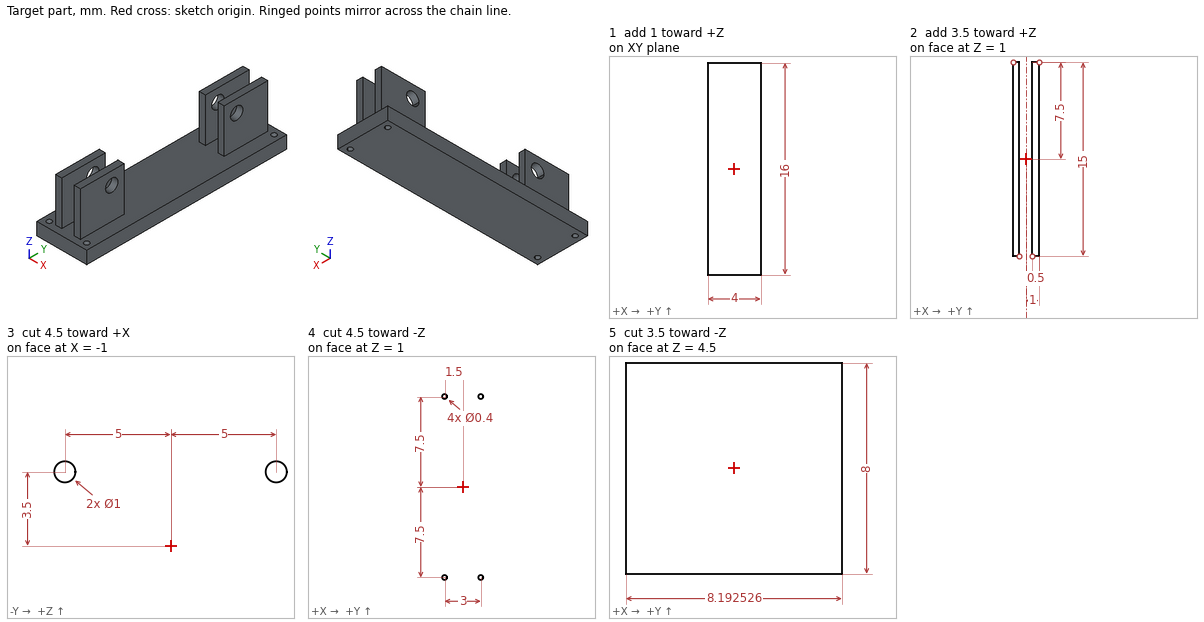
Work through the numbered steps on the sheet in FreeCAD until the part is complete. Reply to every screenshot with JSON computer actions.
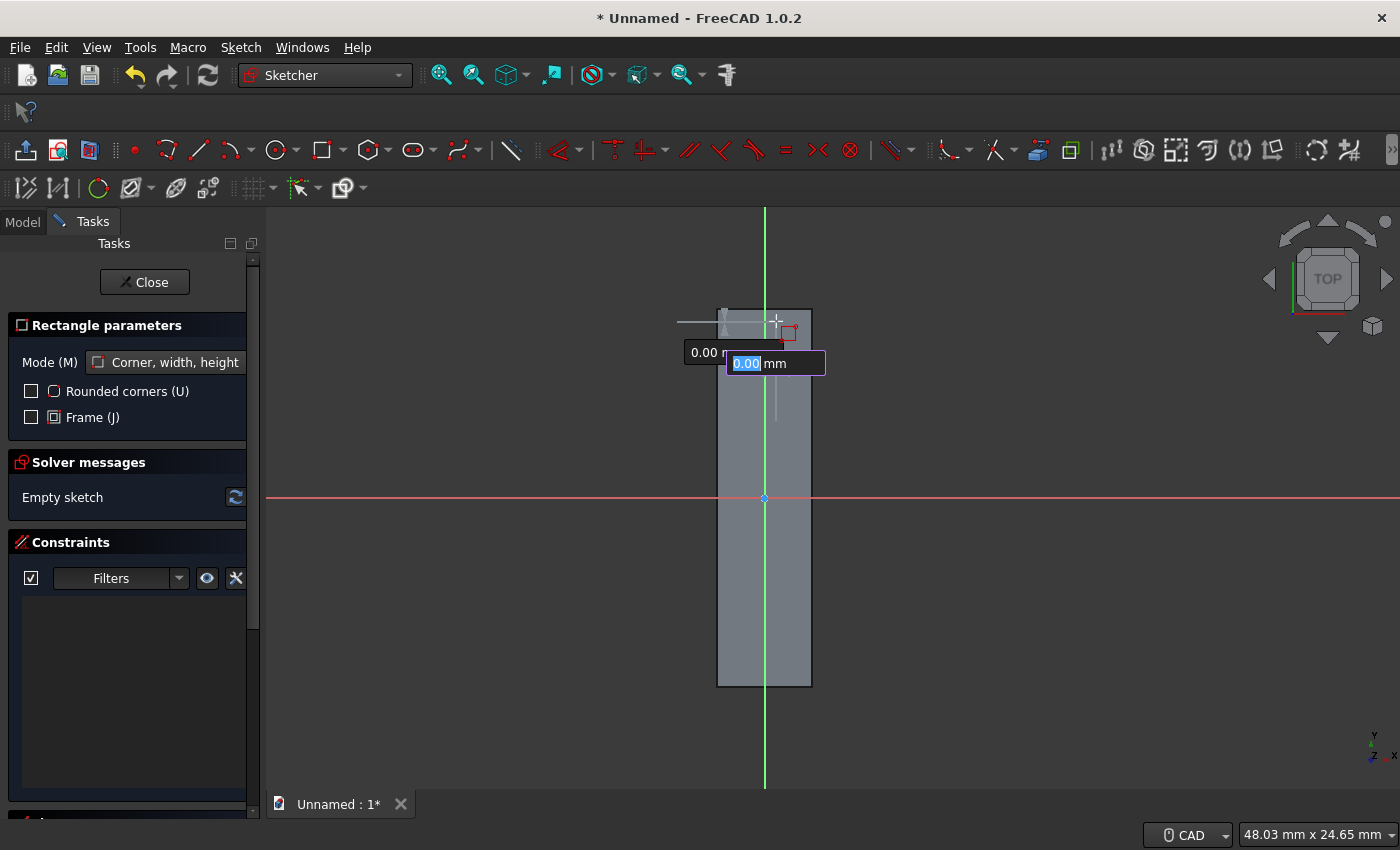
{"action": "left_click", "coordinate": [788, 675]}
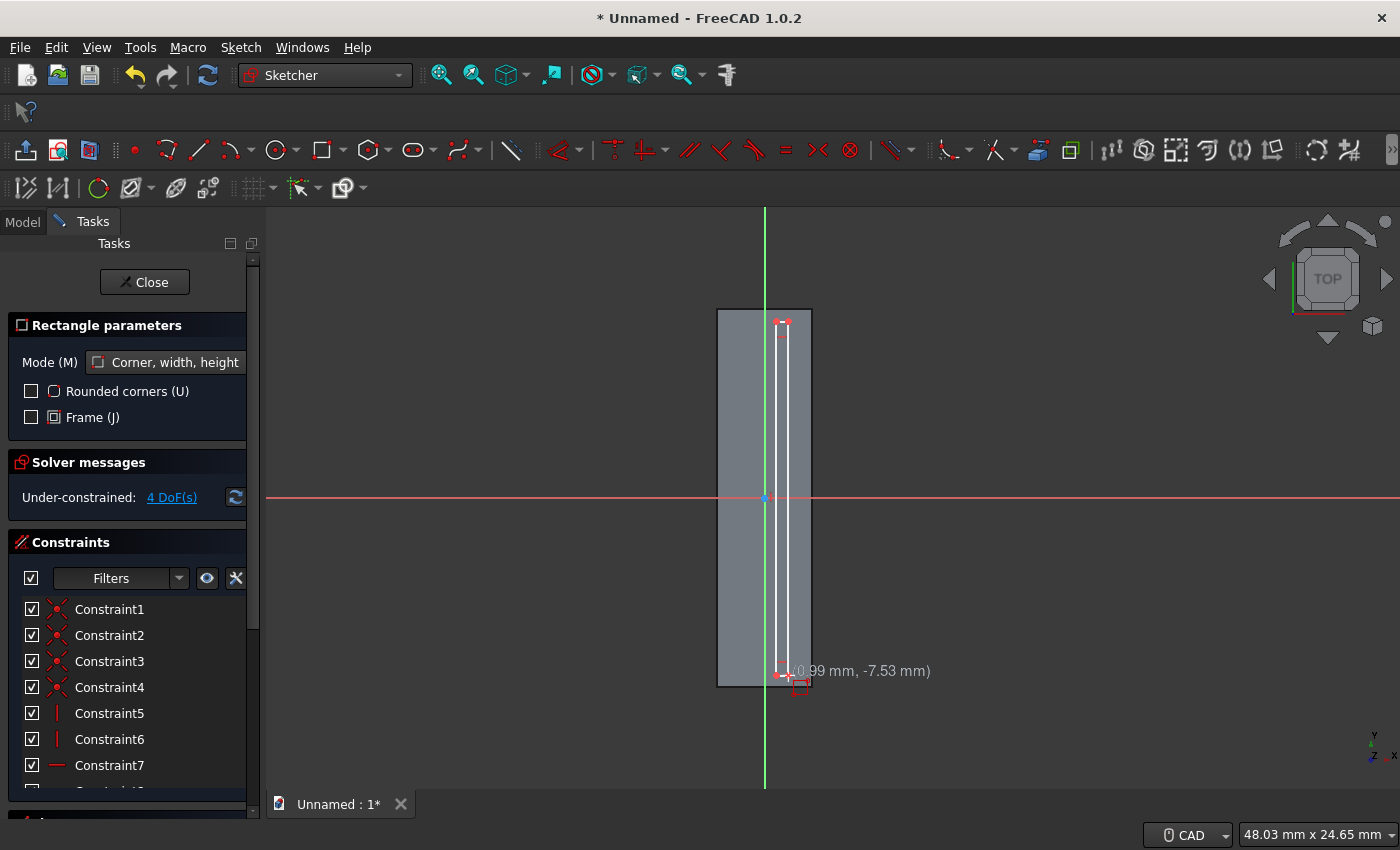
{"action": "scroll", "coordinate": [741, 321], "scroll_direction": "up", "scroll_amount": 2}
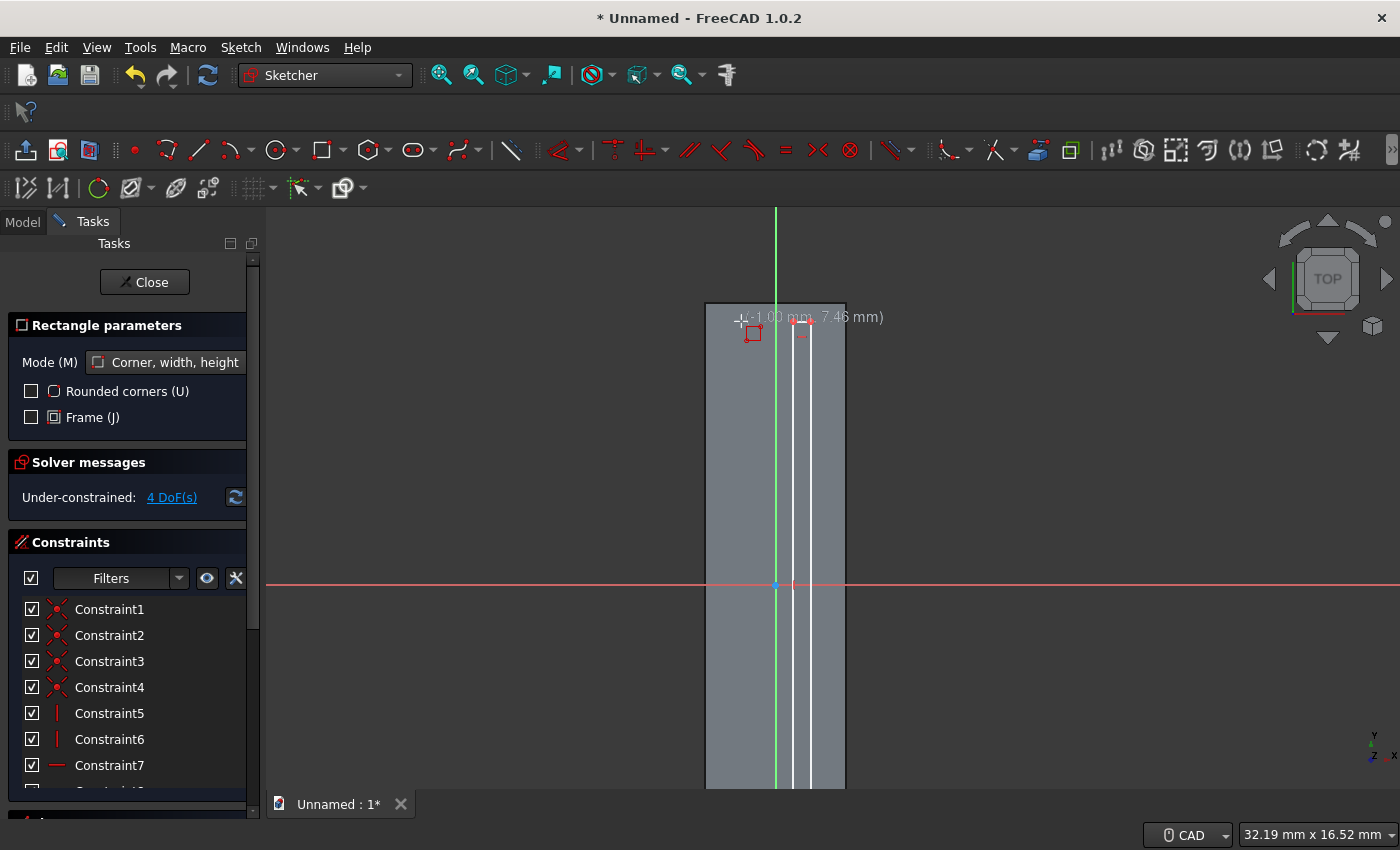
{"action": "left_click", "coordinate": [741, 321]}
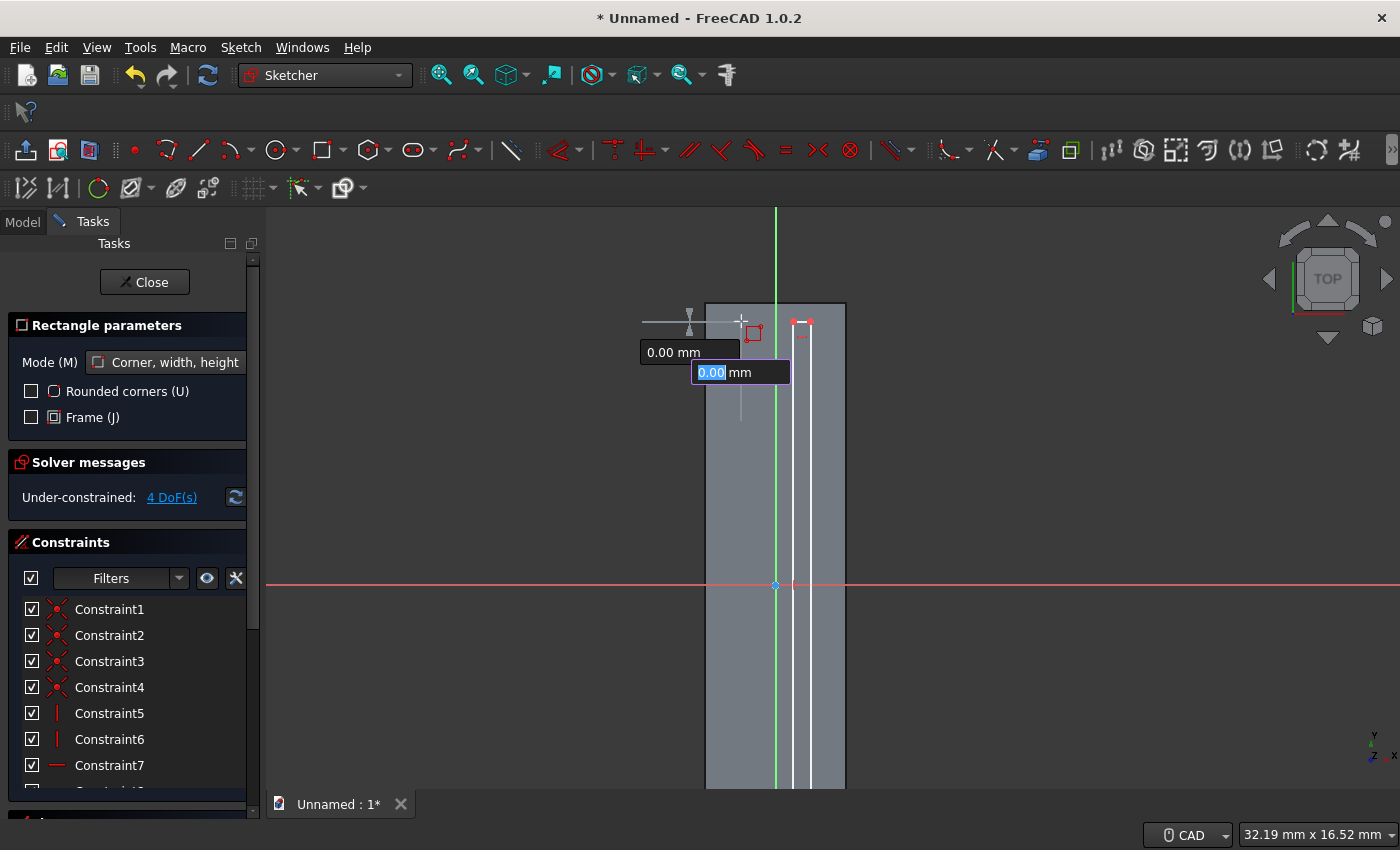
{"action": "scroll", "coordinate": [741, 321], "scroll_direction": "down", "scroll_amount": 2}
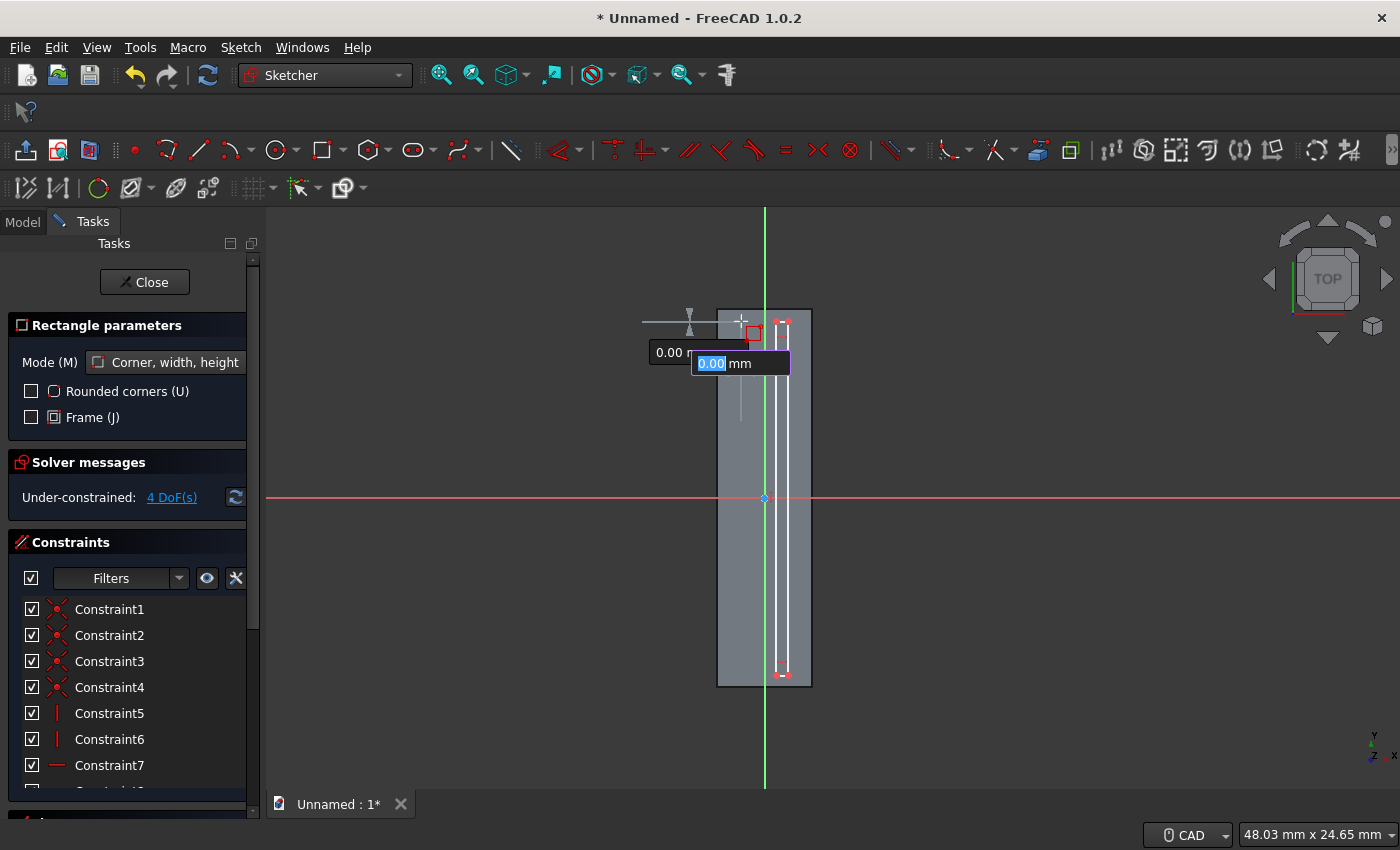
{"action": "scroll", "coordinate": [753, 675], "scroll_direction": "up", "scroll_amount": 2}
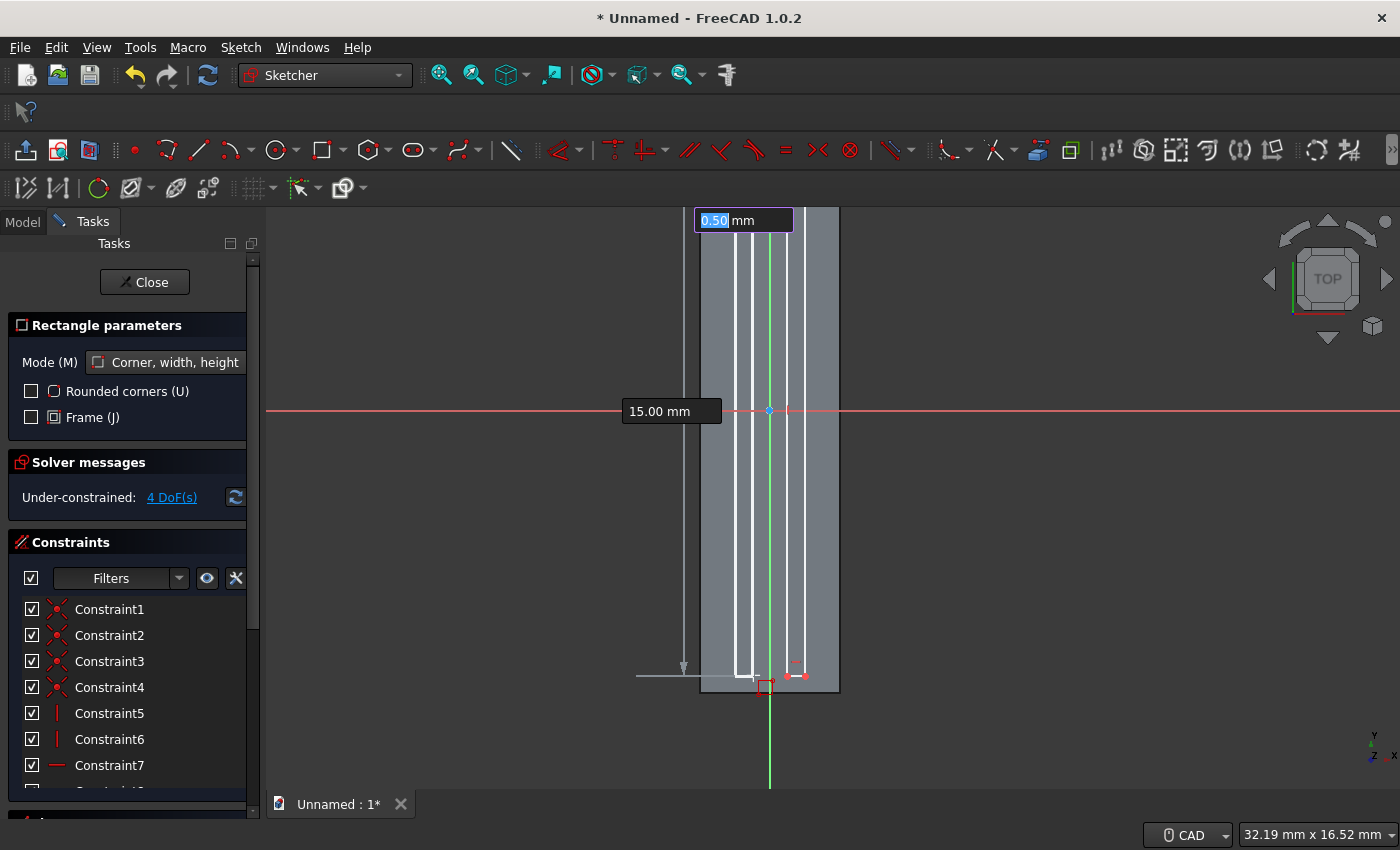
{"action": "left_click", "coordinate": [752, 675]}
{"action": "key", "text": "Escape"}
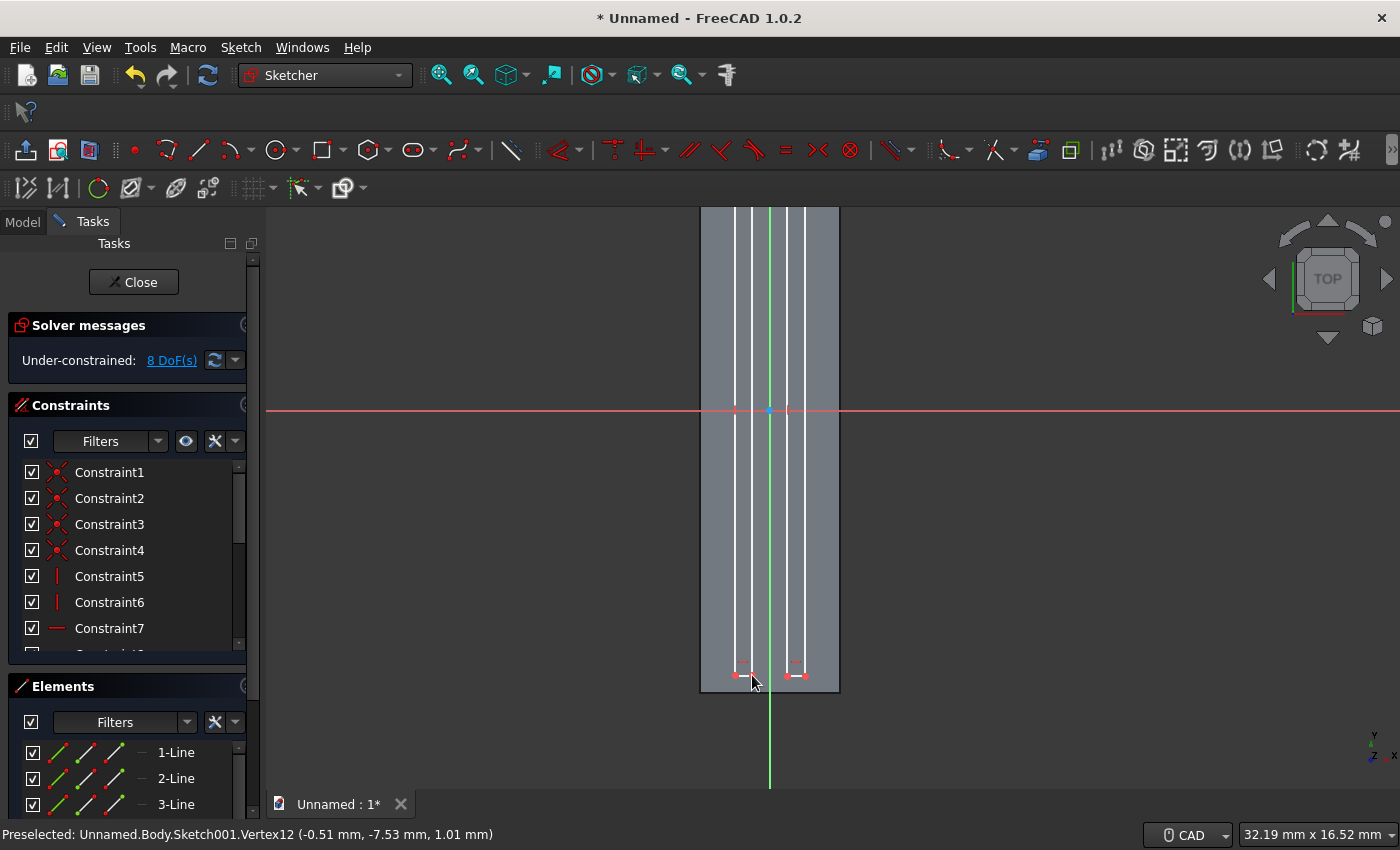
{"action": "scroll", "coordinate": [753, 675], "scroll_direction": "down", "scroll_amount": 2}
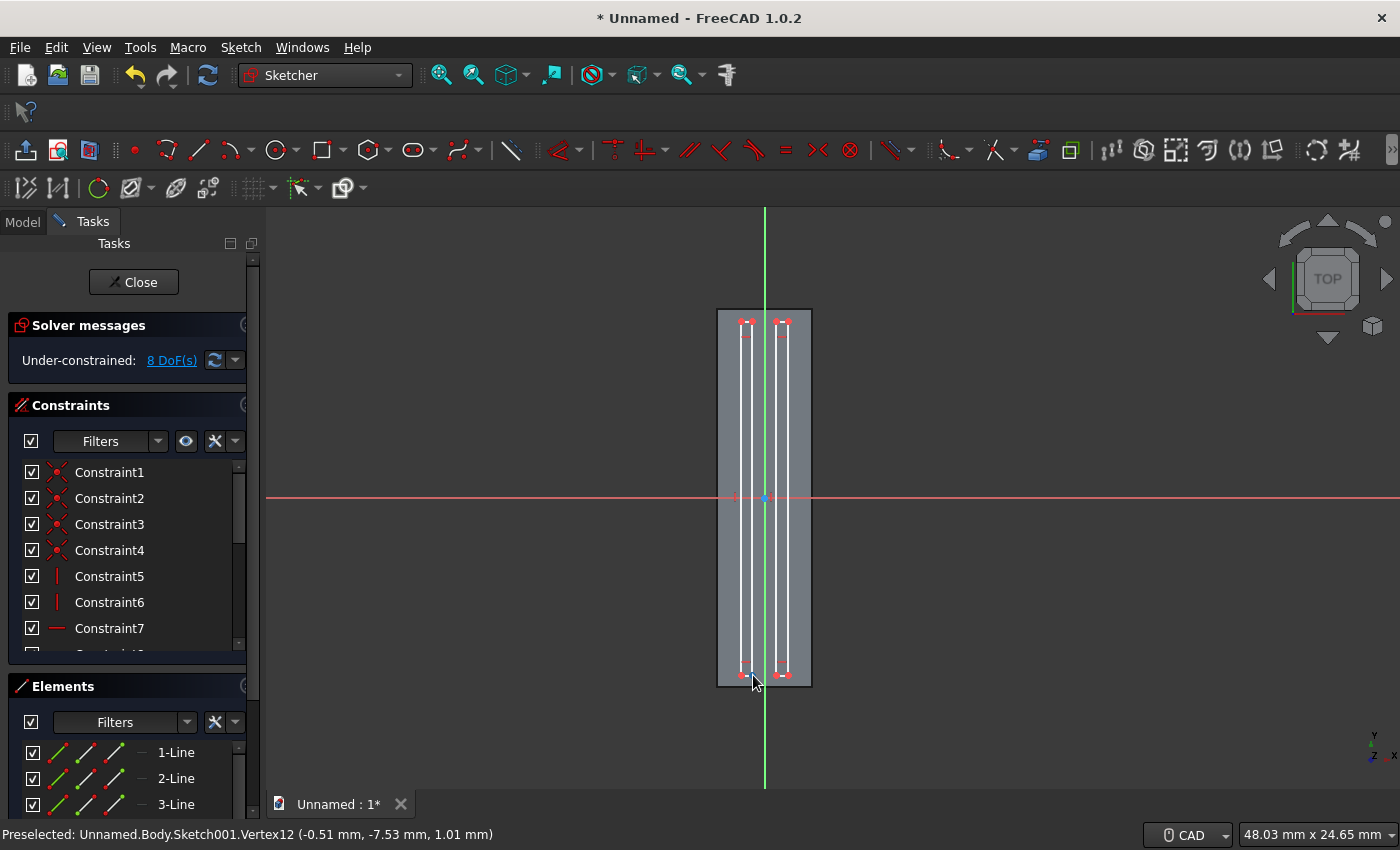
{"action": "left_click", "coordinate": [788, 322]}